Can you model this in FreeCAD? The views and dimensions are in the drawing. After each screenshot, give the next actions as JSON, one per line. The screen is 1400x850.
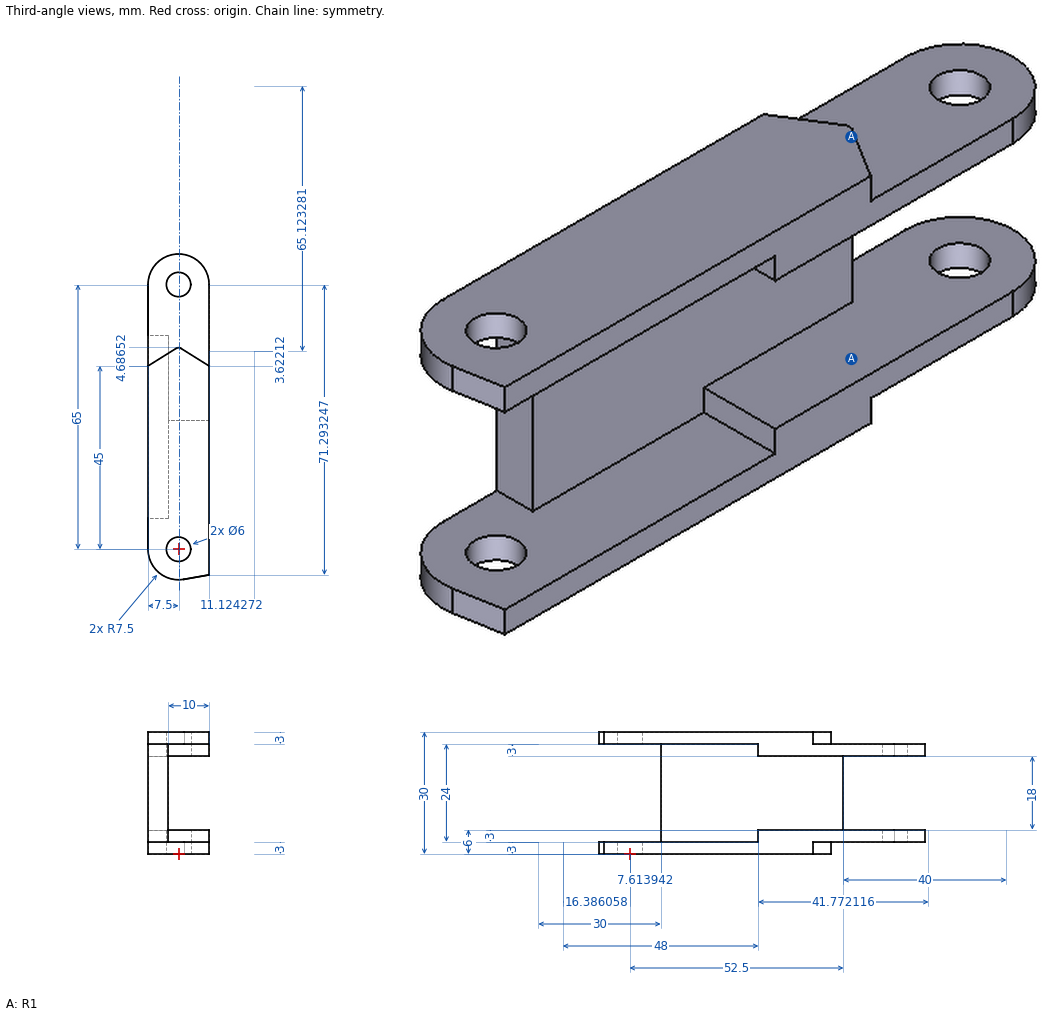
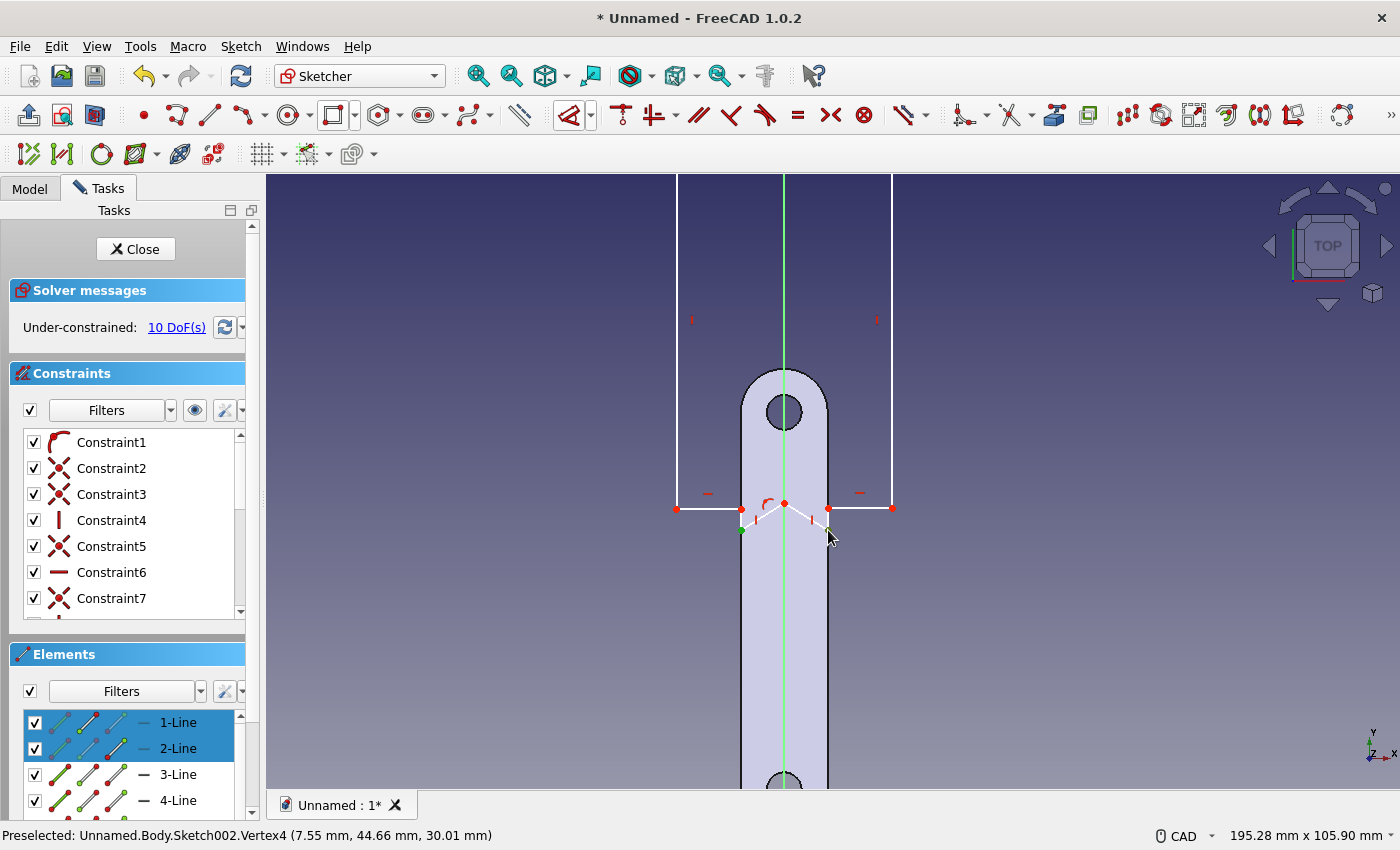
{"action": "left_click", "coordinate": [784, 721]}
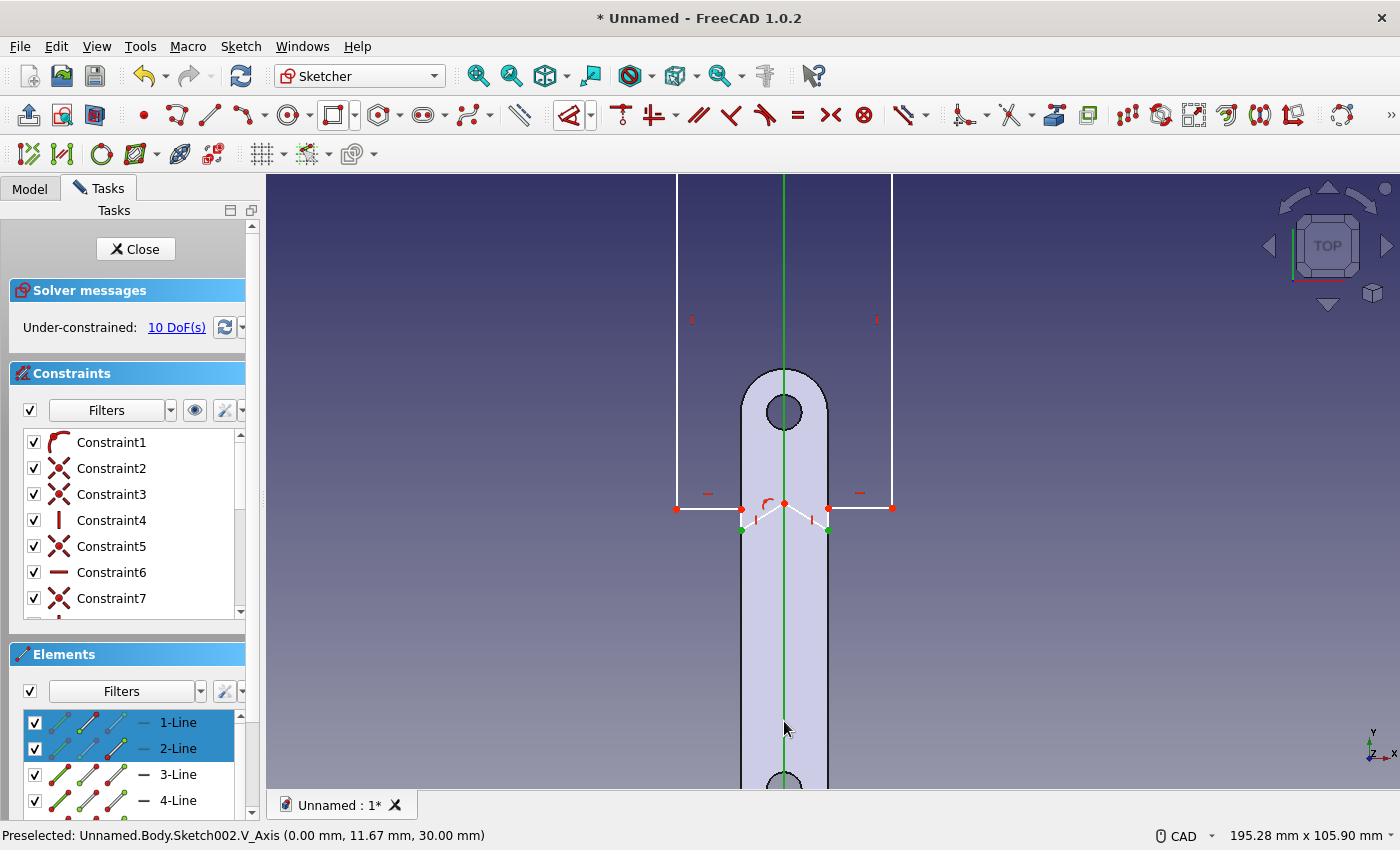
{"action": "left_click", "coordinate": [831, 116]}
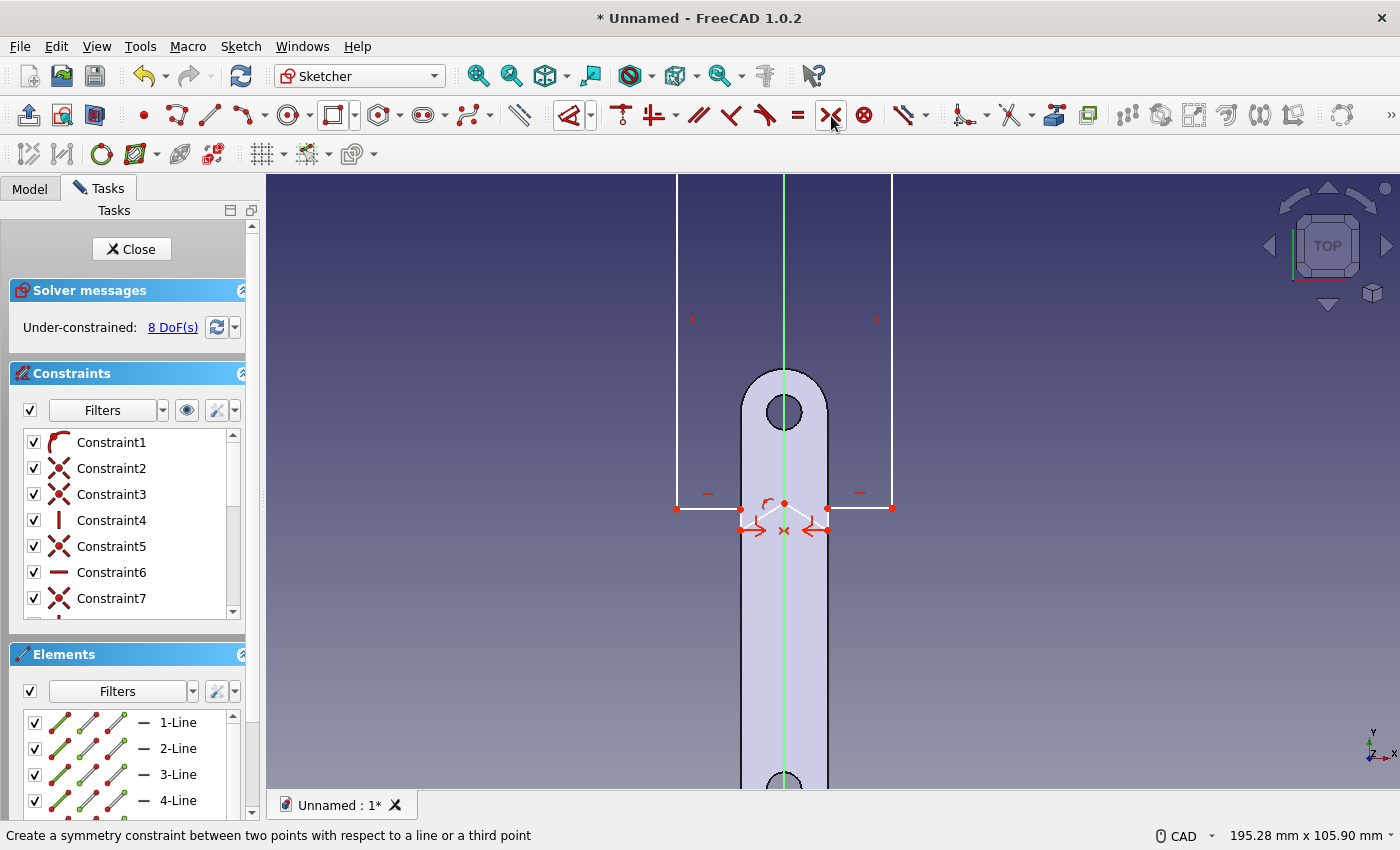
{"action": "left_click", "coordinate": [892, 508]}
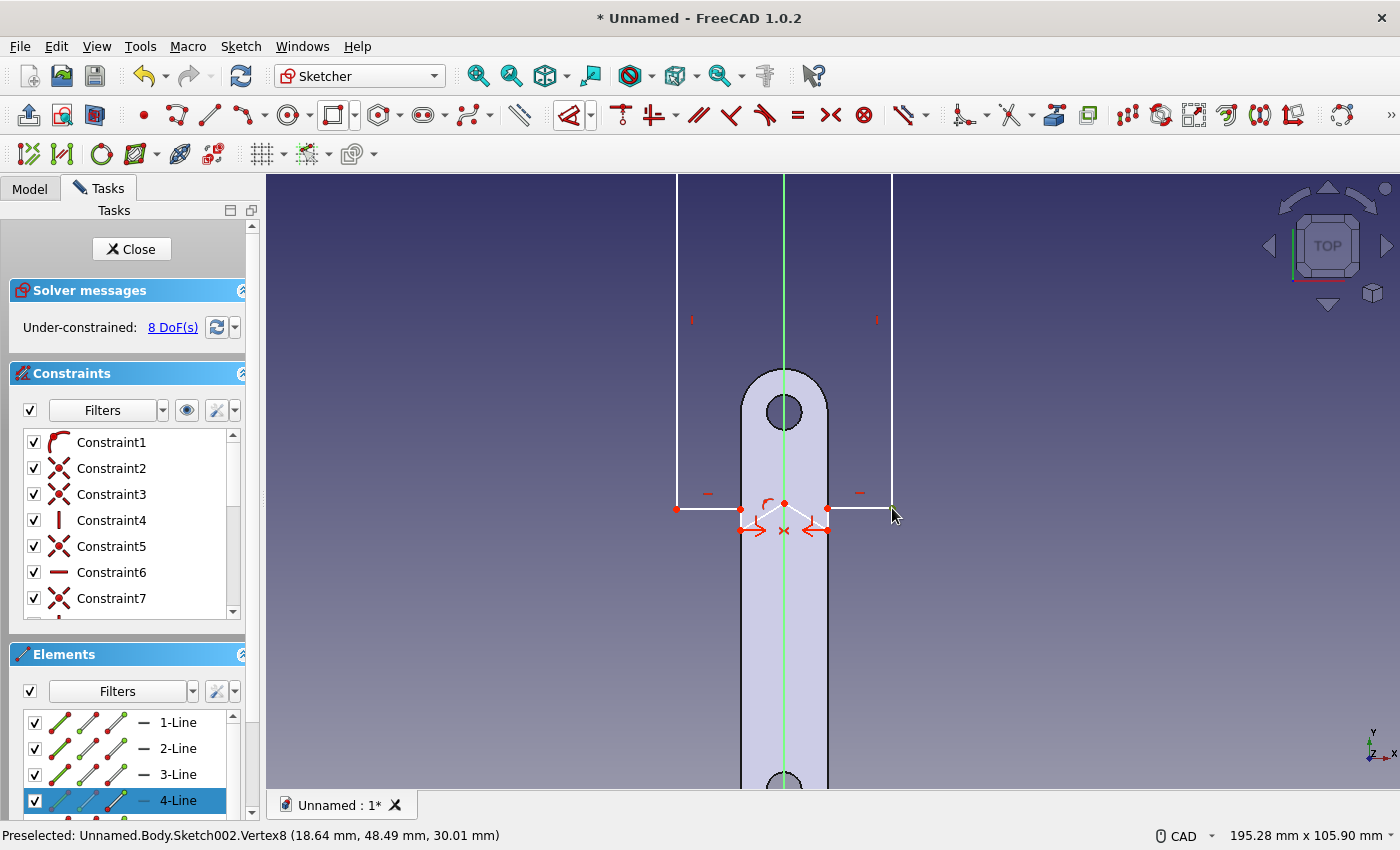
{"action": "left_click", "coordinate": [677, 509]}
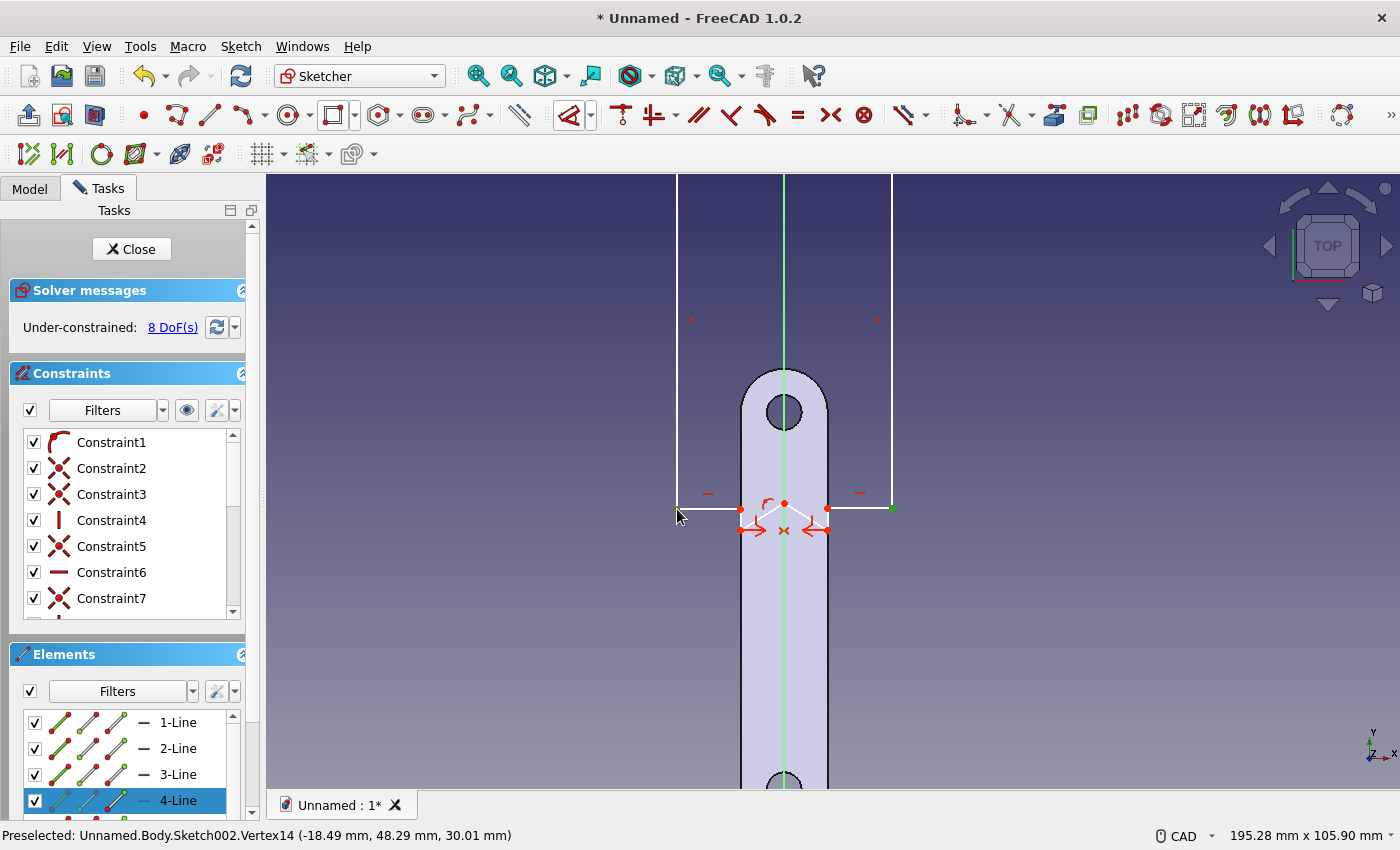
{"action": "left_click", "coordinate": [784, 721]}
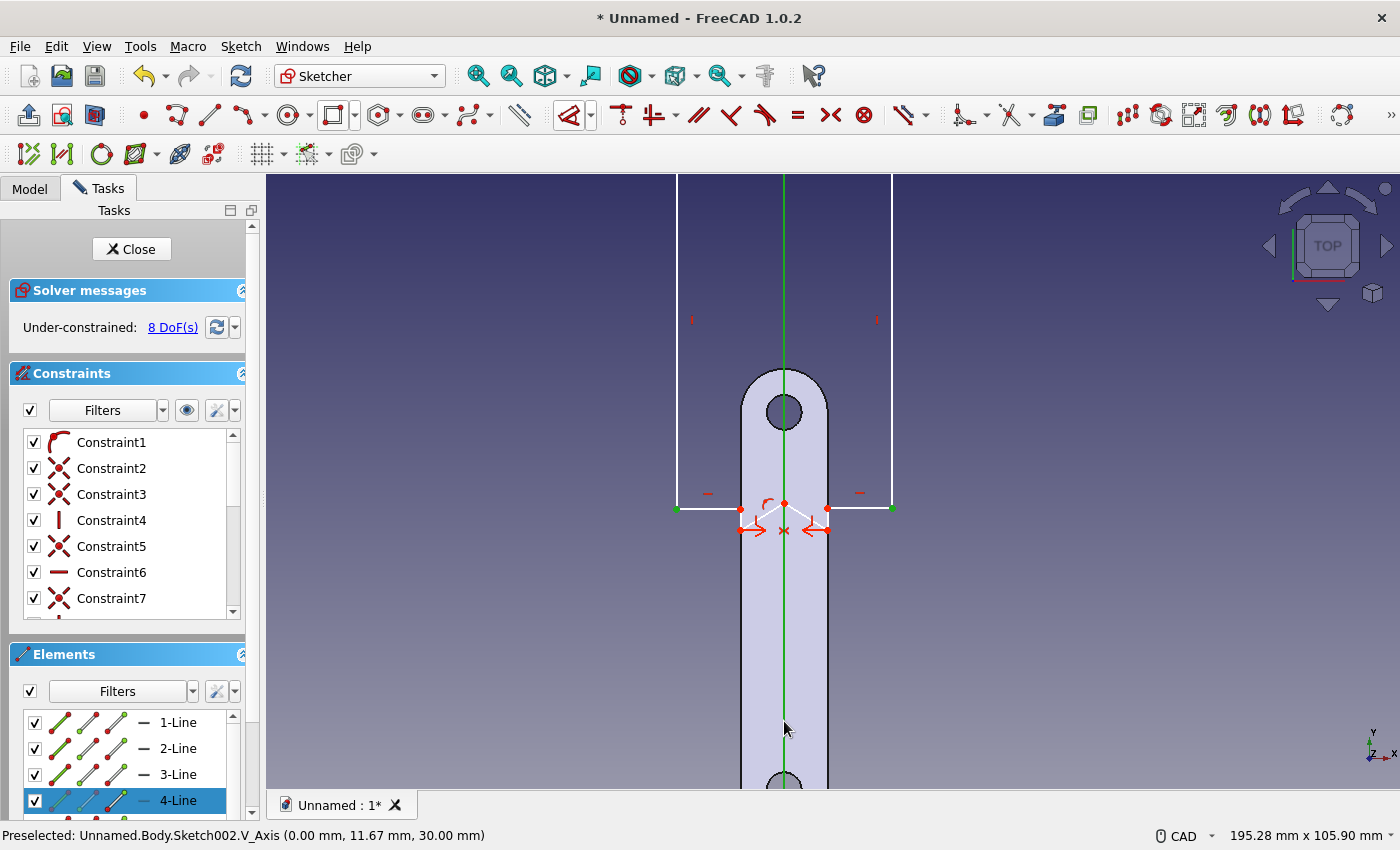
{"action": "left_click", "coordinate": [831, 116]}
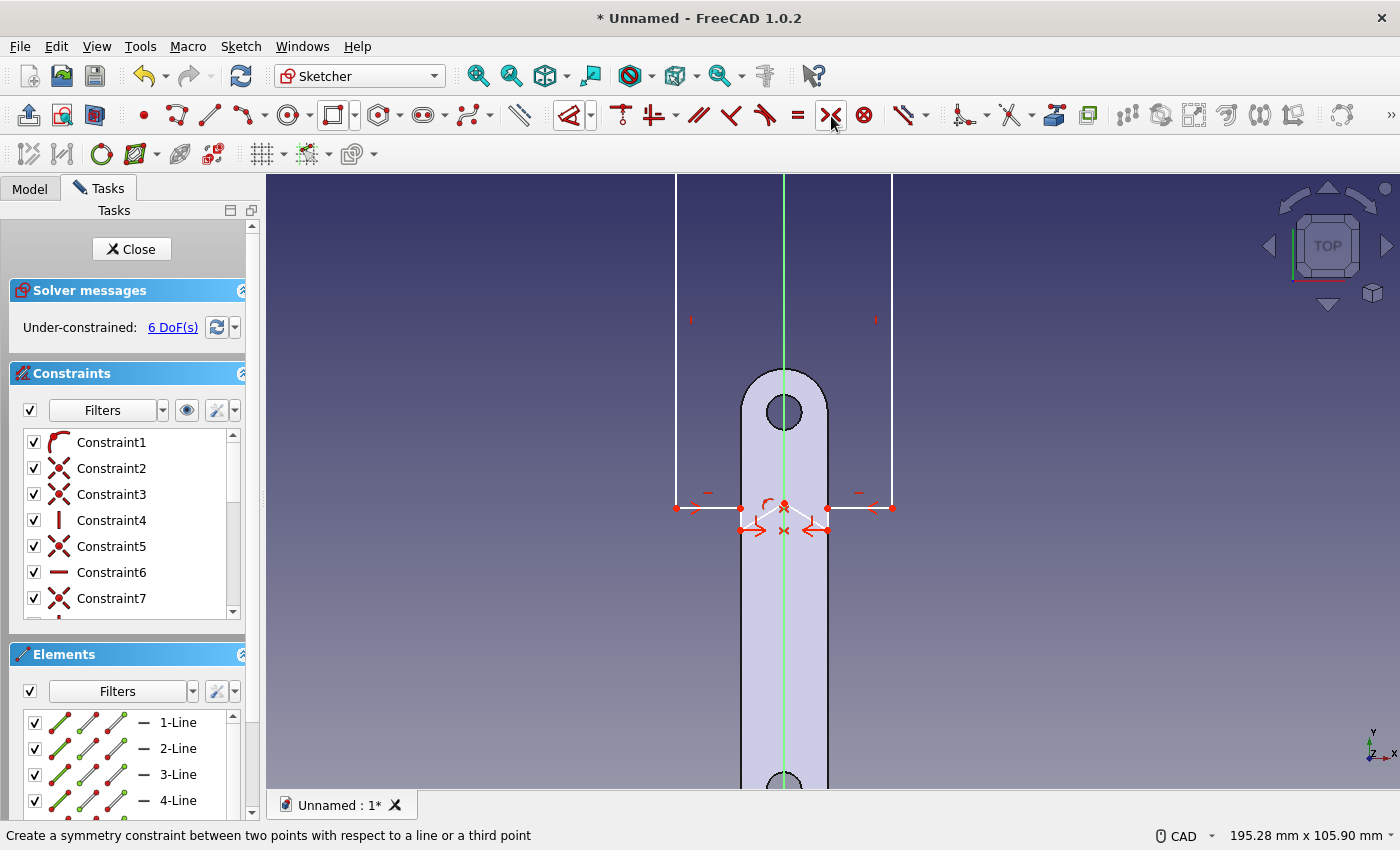
{"action": "left_click", "coordinate": [741, 530]}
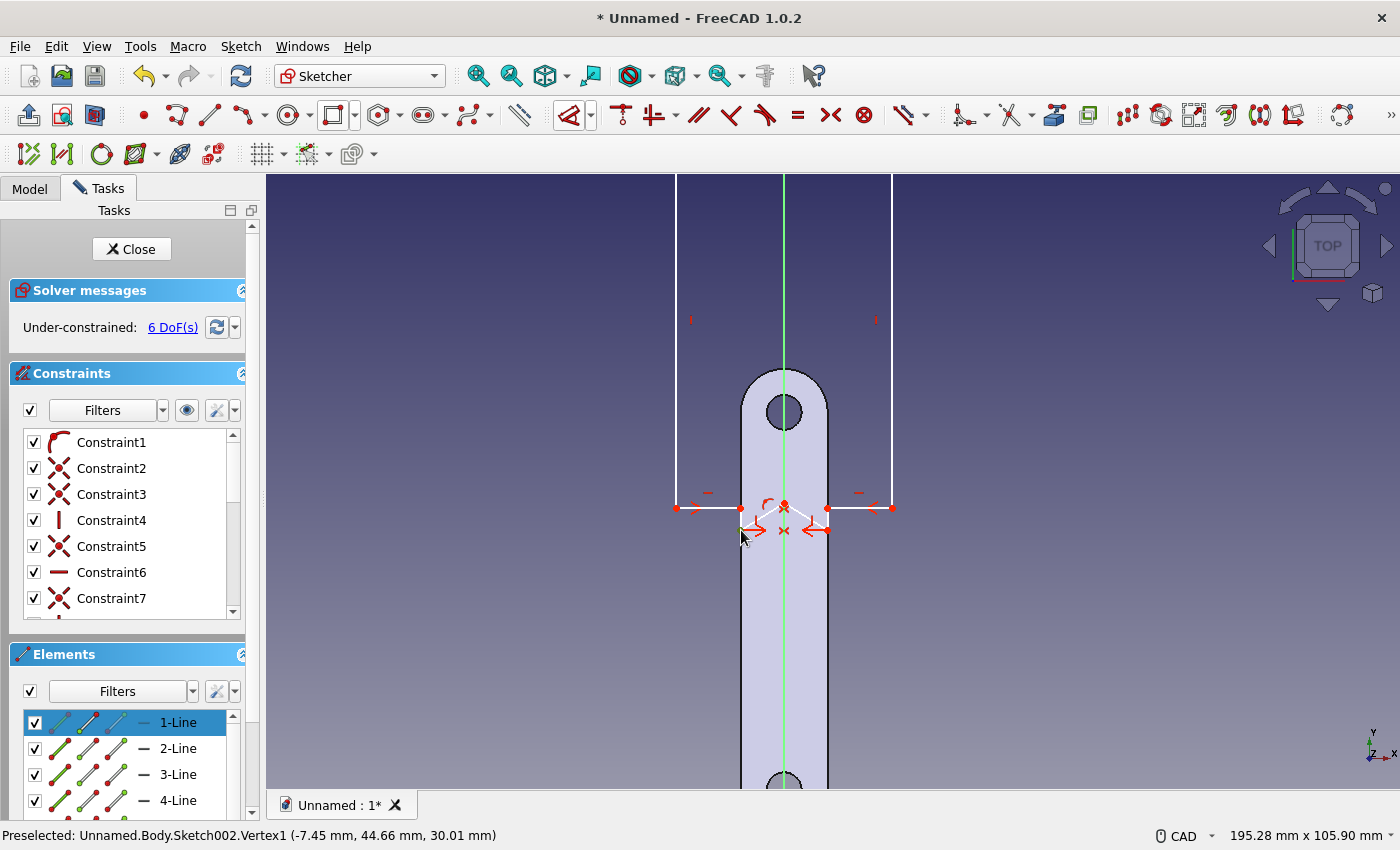
{"action": "key", "text": "i"}